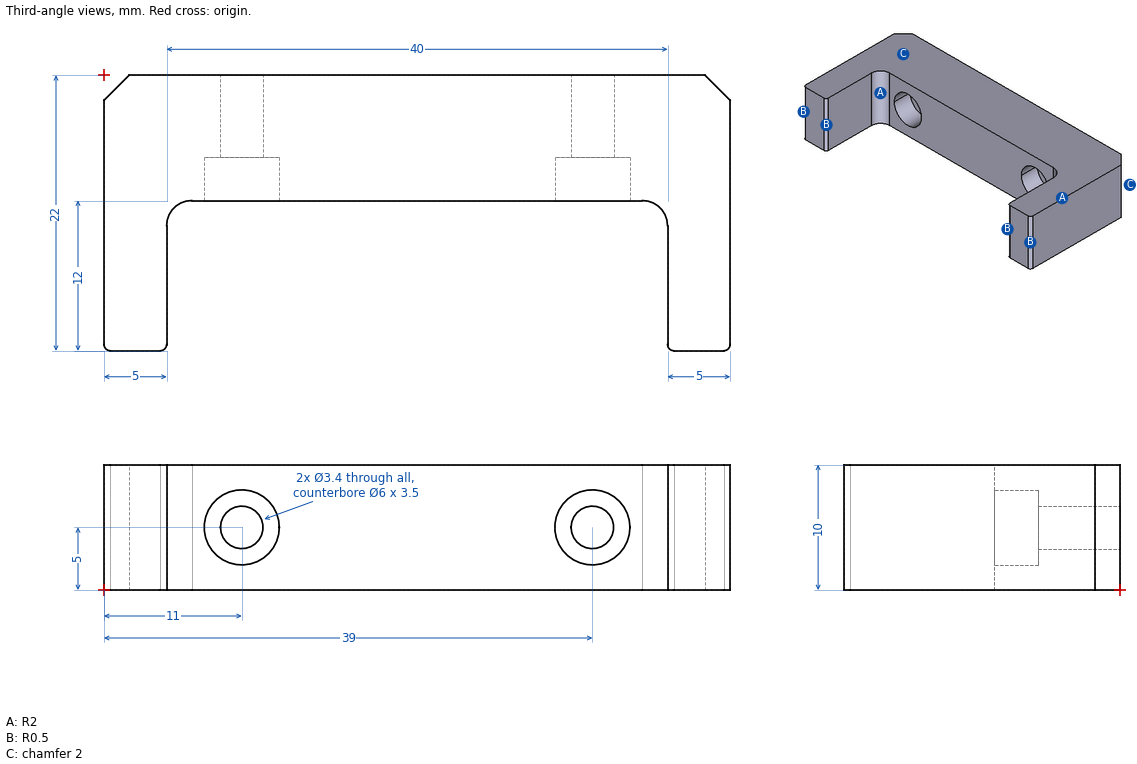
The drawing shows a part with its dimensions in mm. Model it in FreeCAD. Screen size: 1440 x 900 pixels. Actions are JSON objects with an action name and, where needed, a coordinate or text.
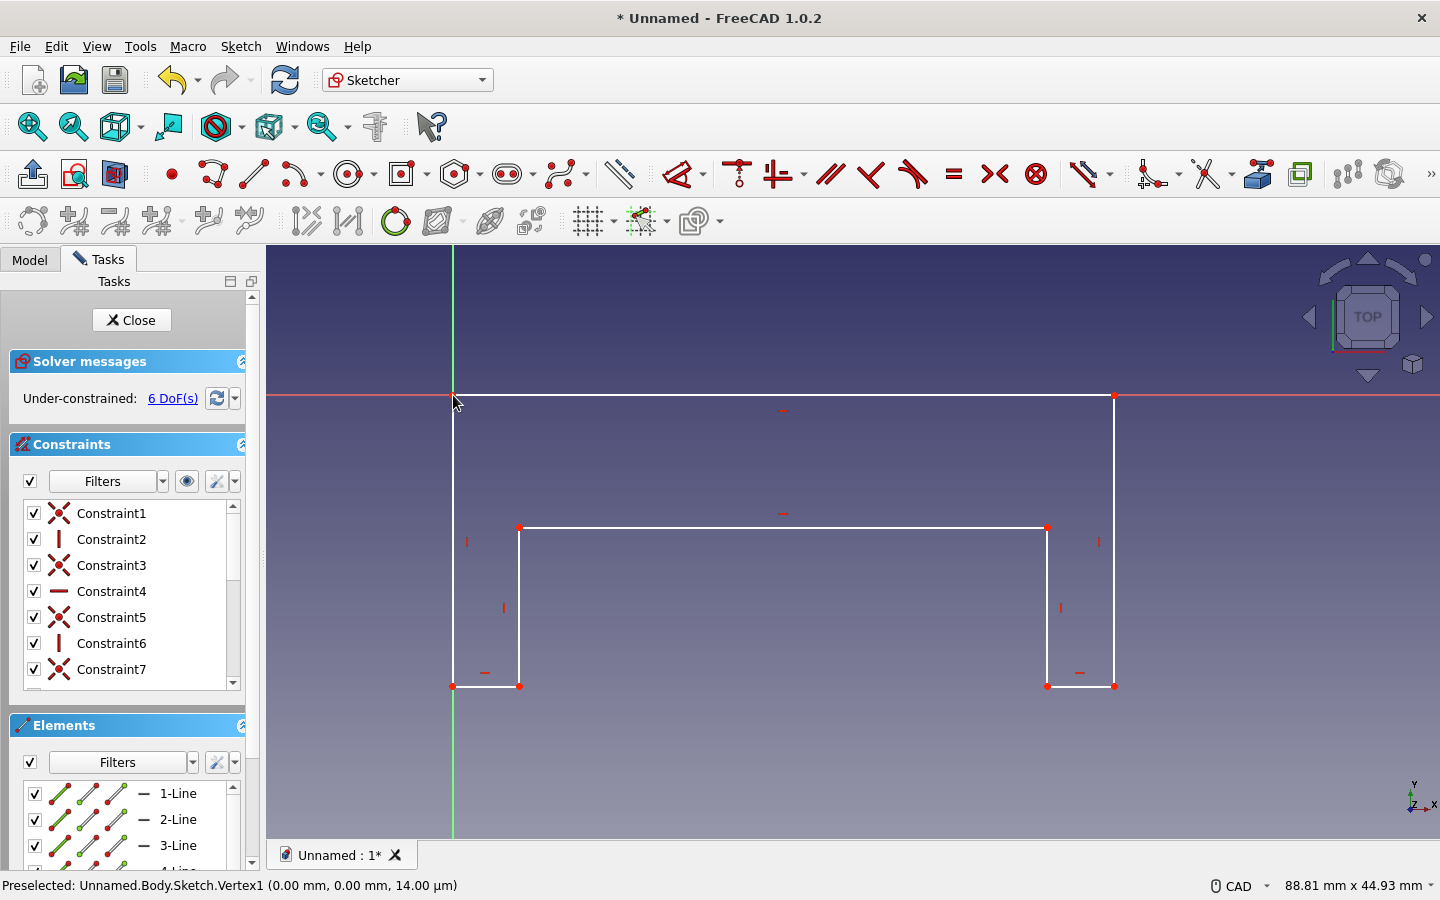
{"action": "left_click", "coordinate": [676, 174]}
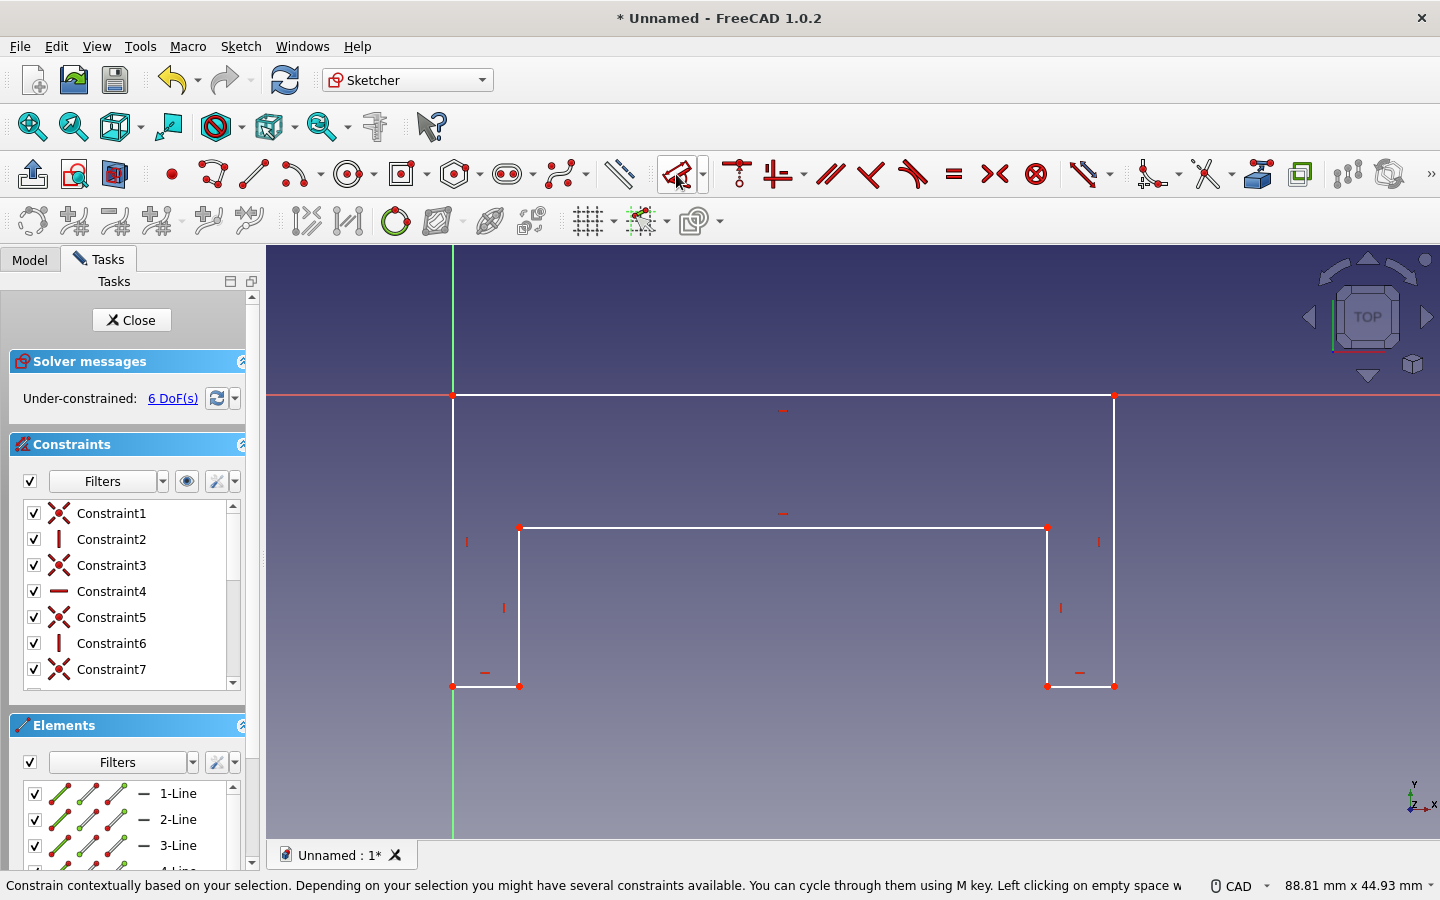
{"action": "left_click", "coordinate": [472, 687]}
{"action": "left_click", "coordinate": [486, 721]}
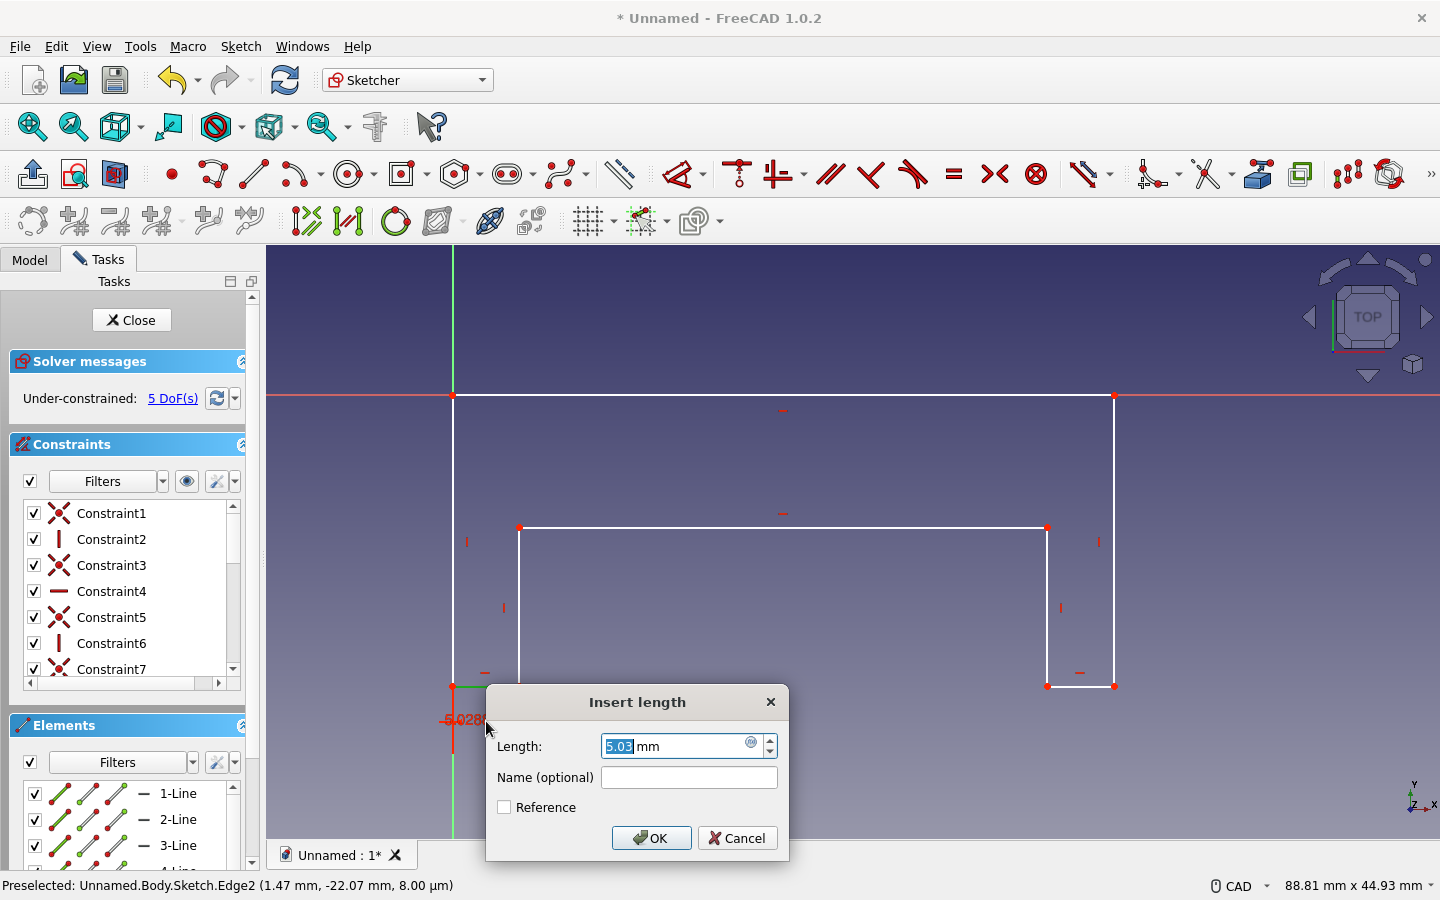
{"action": "type", "text": "5"}
{"action": "key", "text": "Return"}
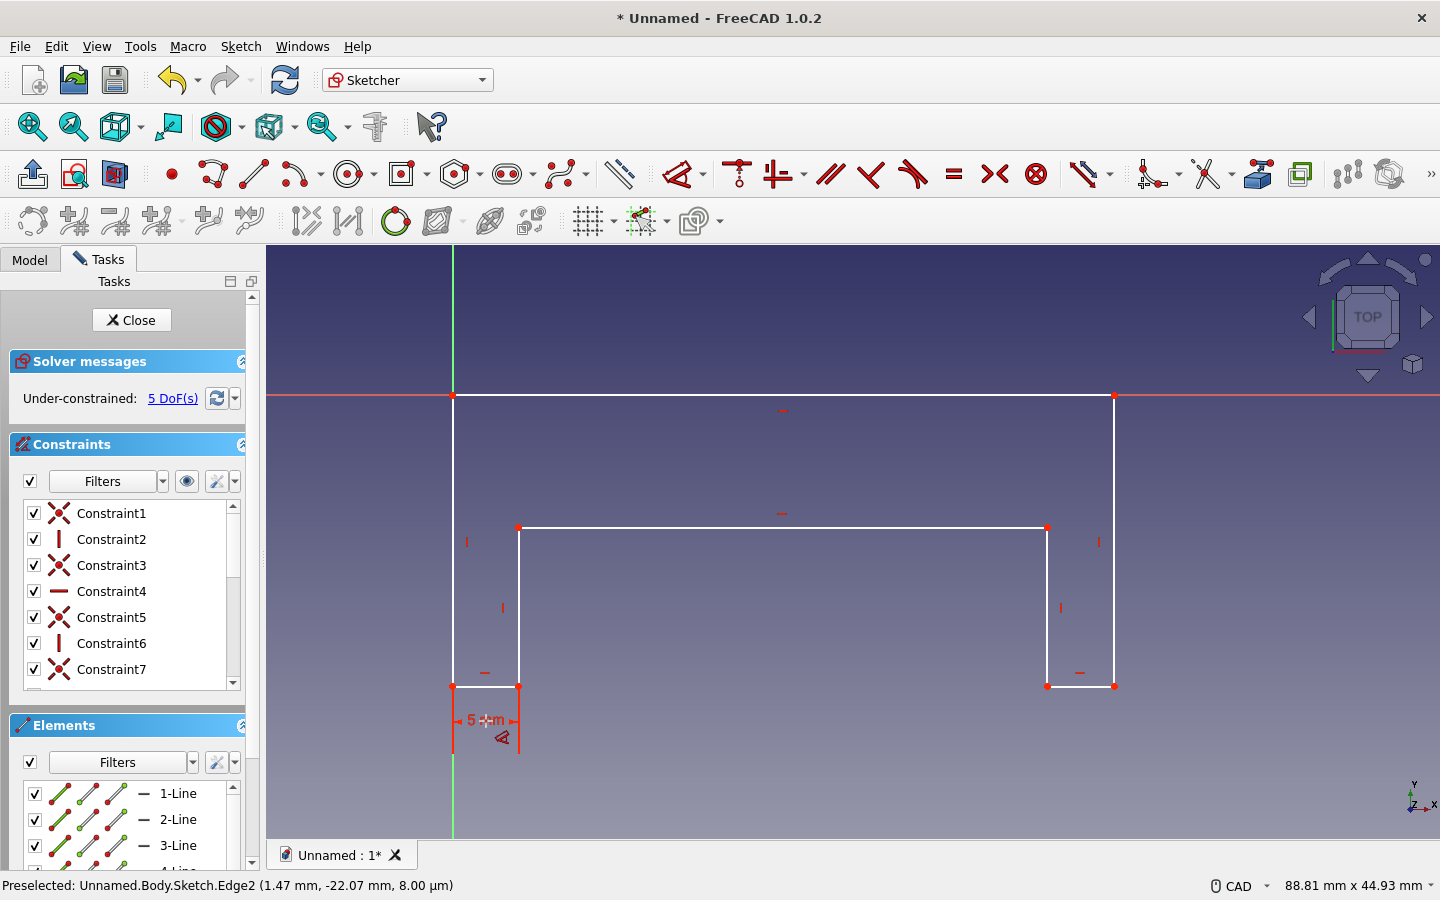
{"action": "left_click", "coordinate": [1067, 687]}
{"action": "left_click", "coordinate": [1081, 721]}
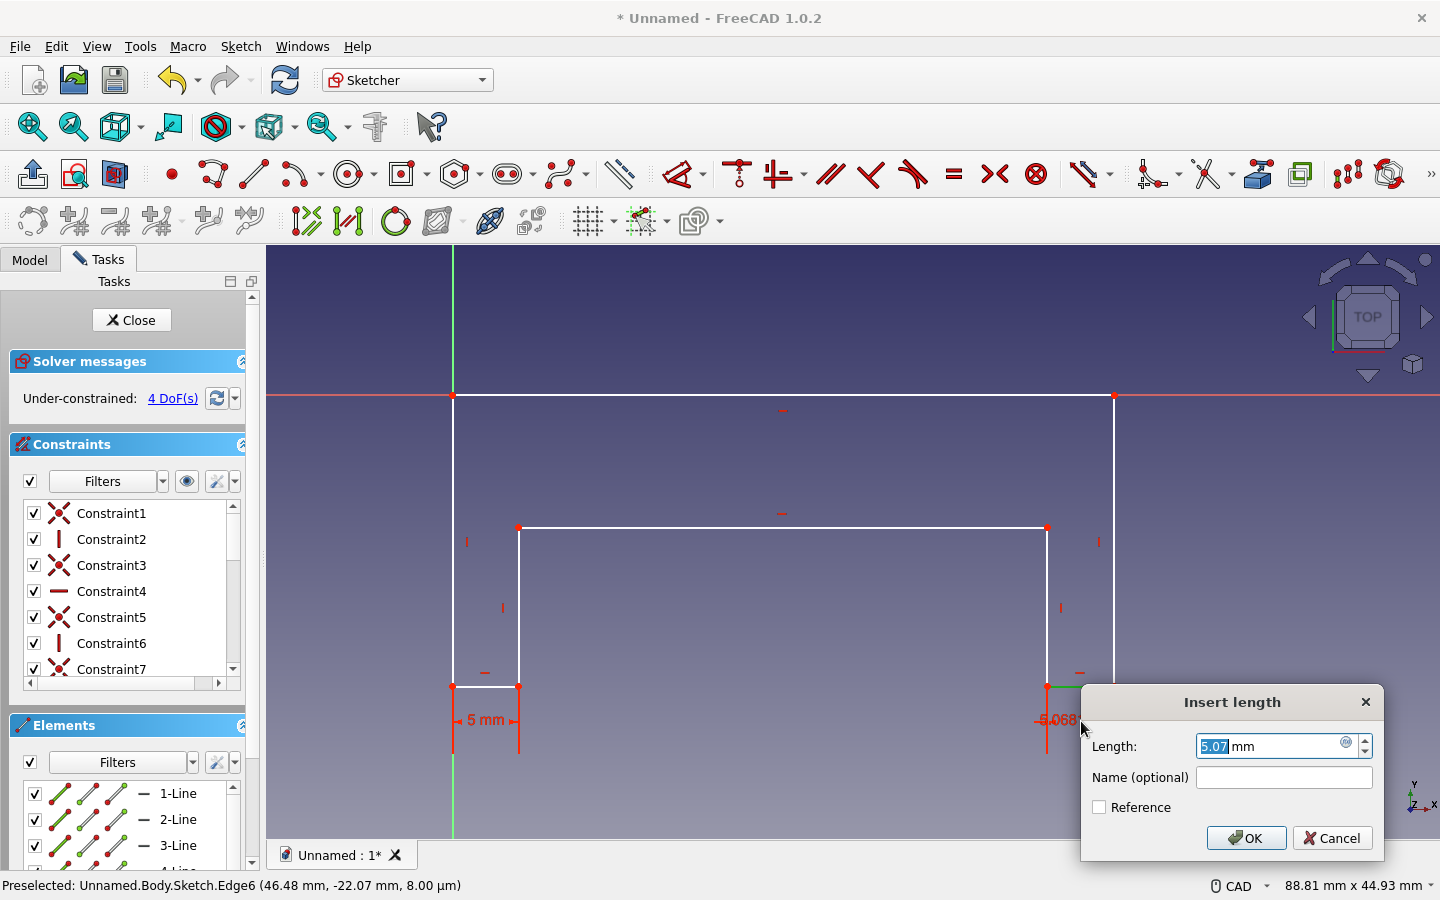
{"action": "type", "text": "5"}
{"action": "key", "text": "Return"}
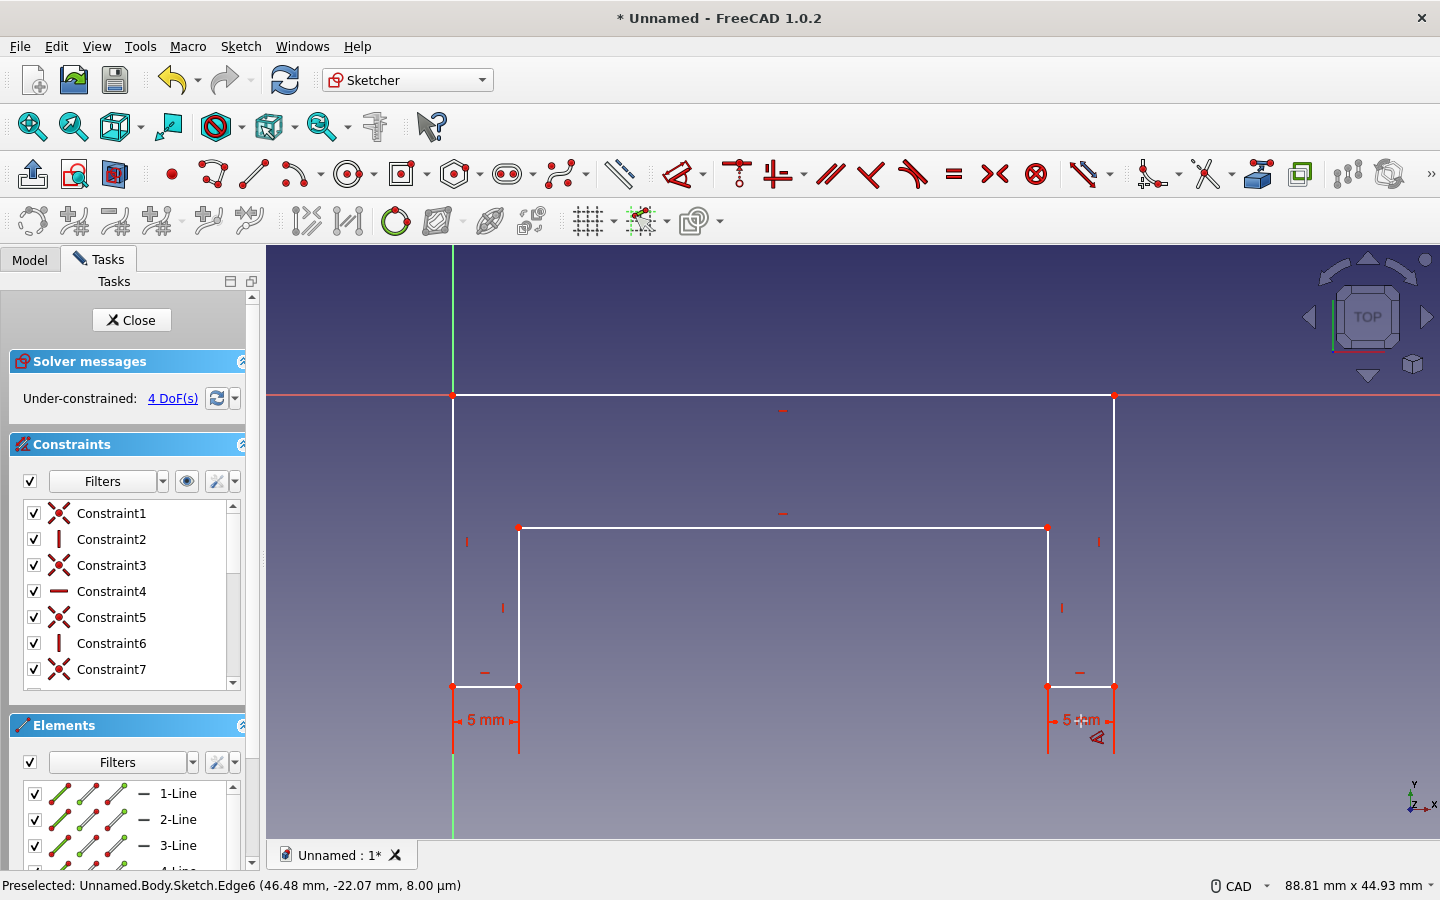
{"action": "left_click", "coordinate": [453, 483]}
{"action": "left_click", "coordinate": [419, 541]}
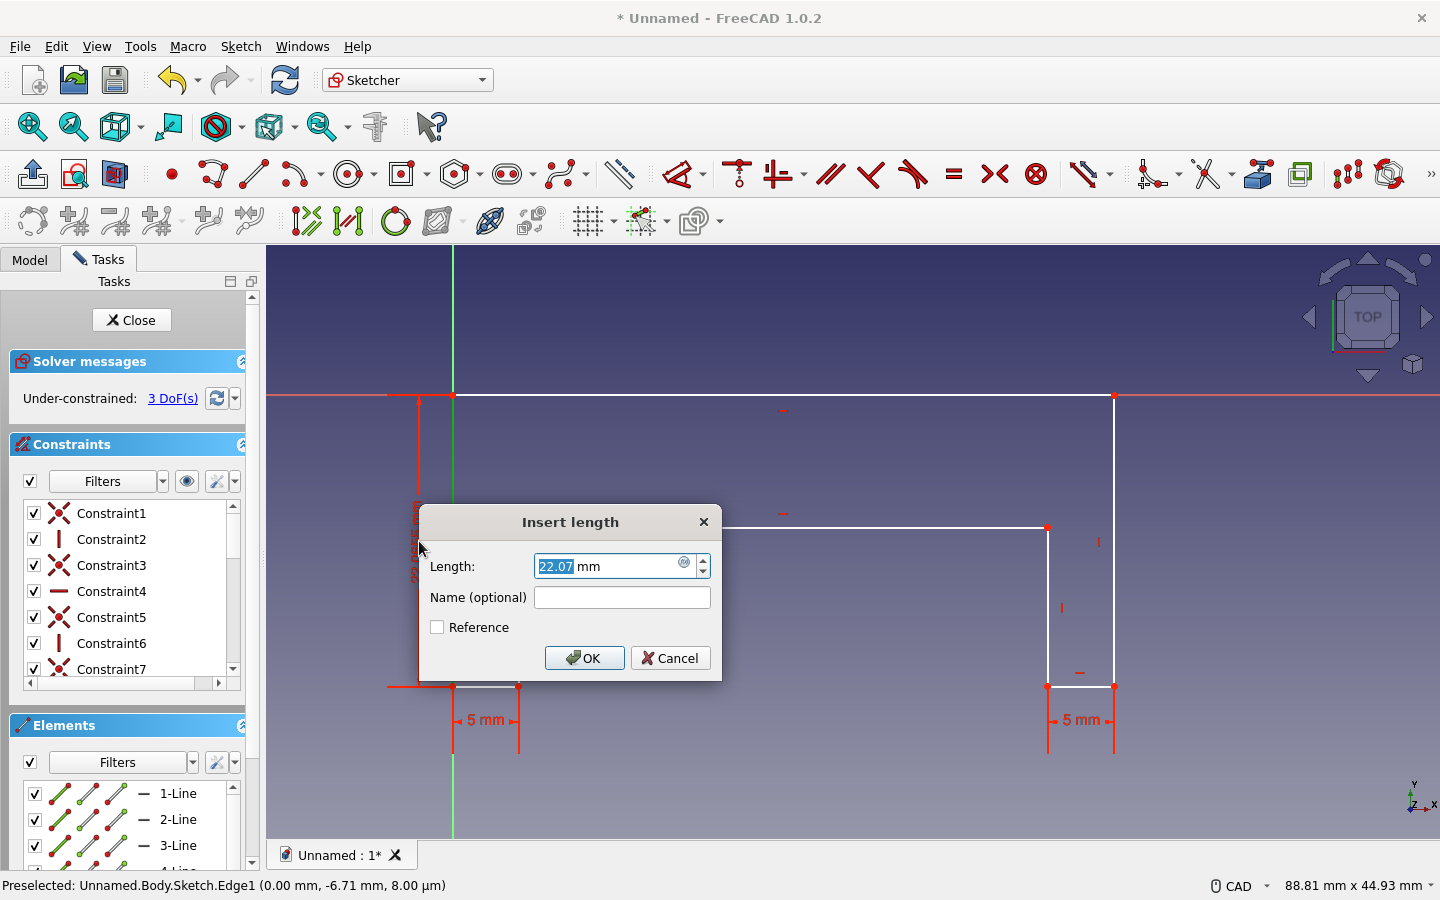
{"action": "type", "text": "22"}
{"action": "key", "text": "Return"}